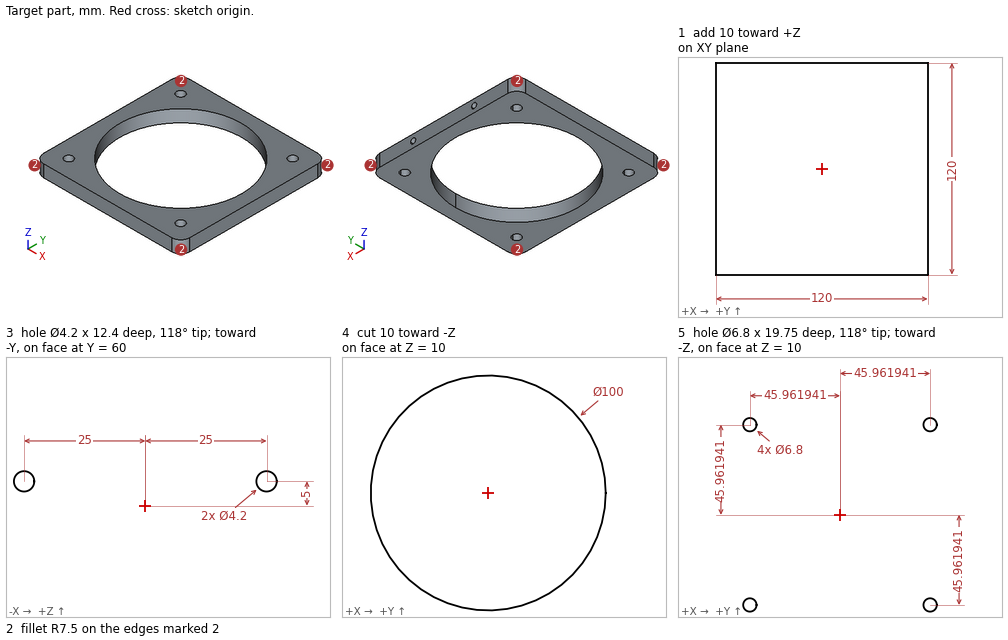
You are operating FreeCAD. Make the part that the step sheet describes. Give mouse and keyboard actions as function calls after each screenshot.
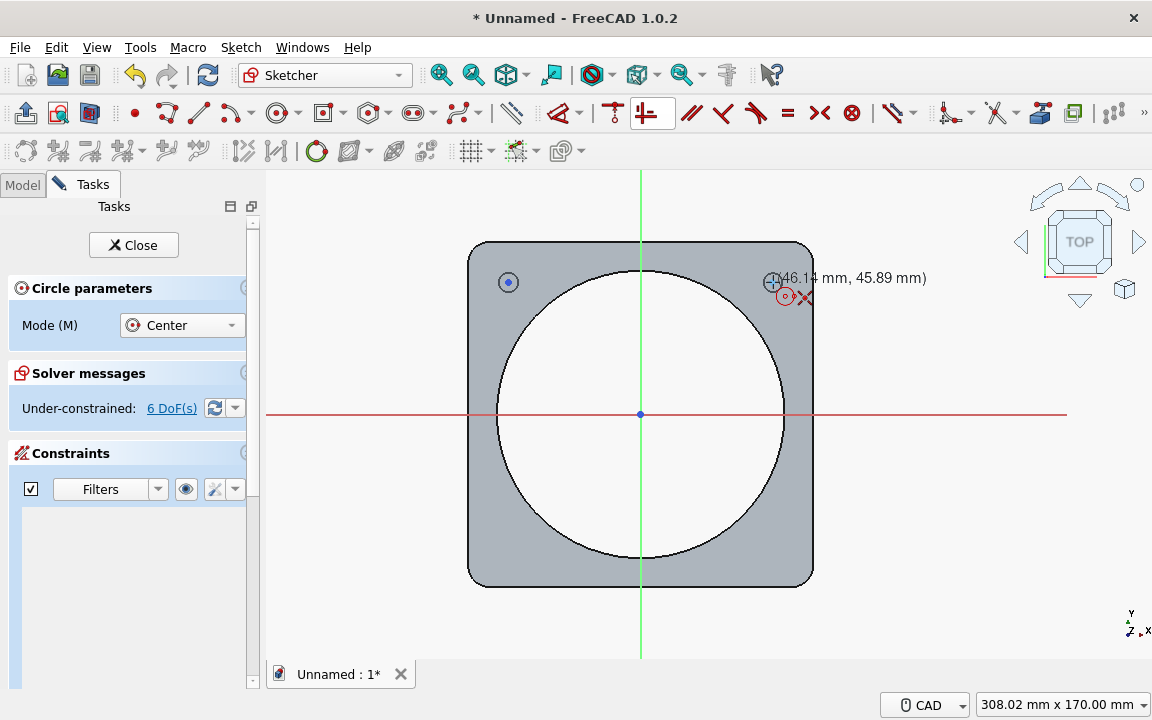
scroll(773, 547, up, 5)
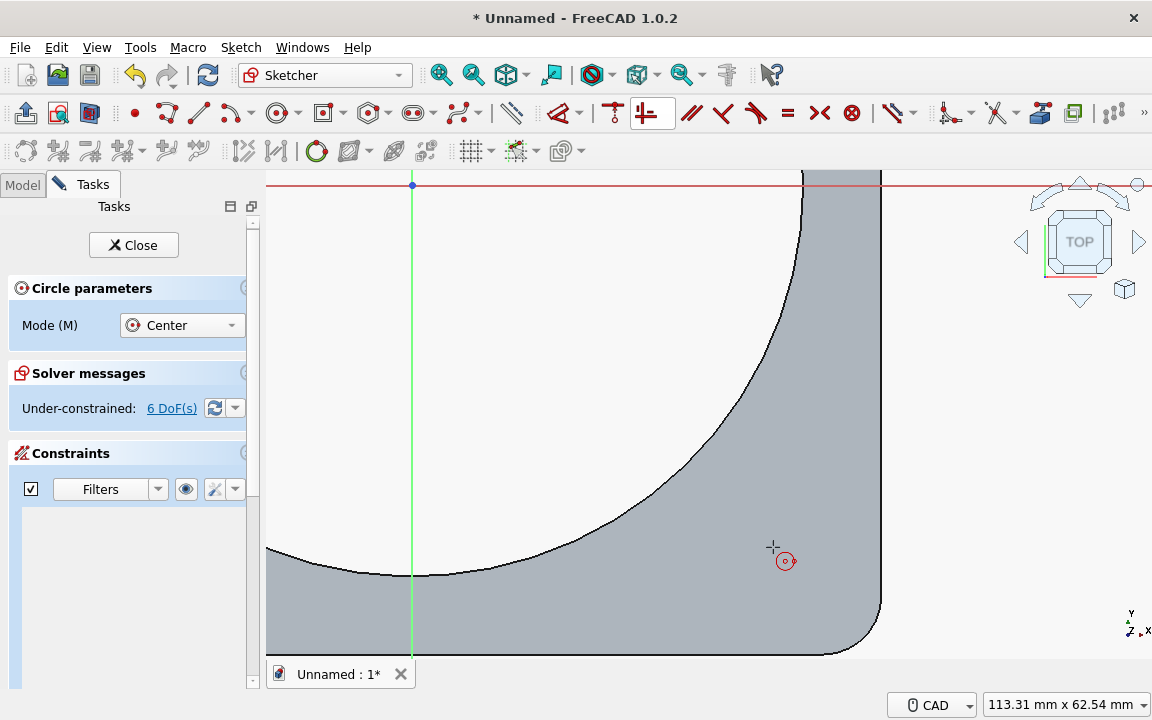
click(772, 545)
click(790, 526)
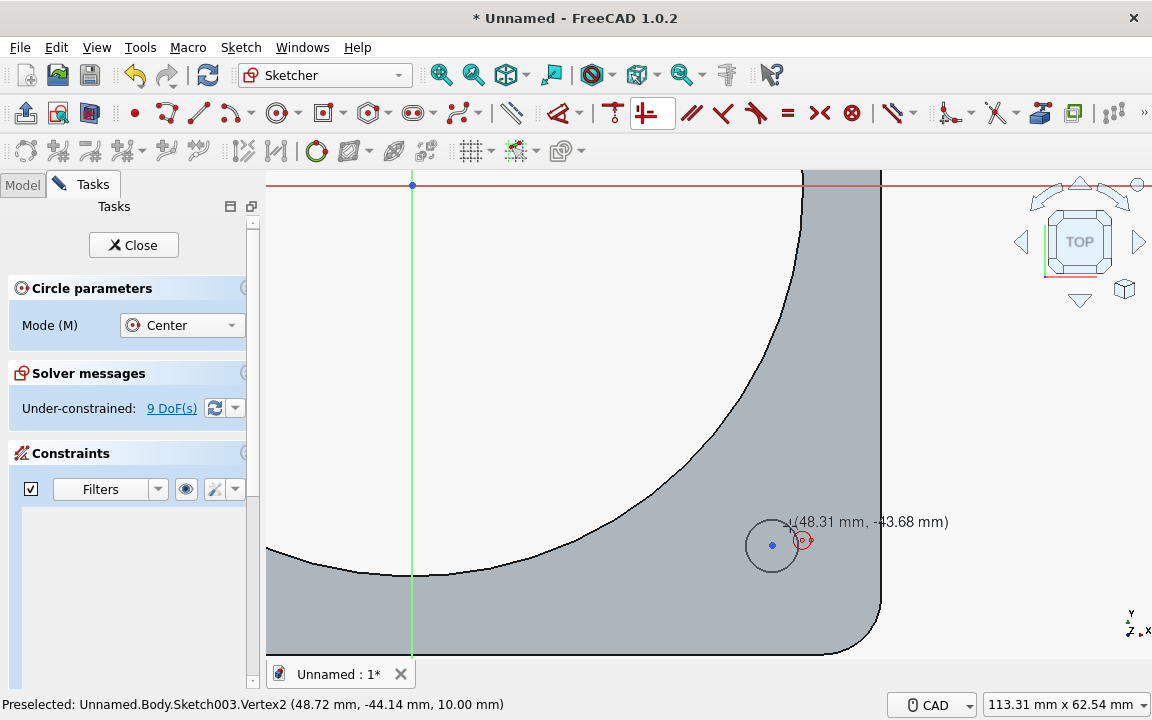
scroll(773, 548, down, 5)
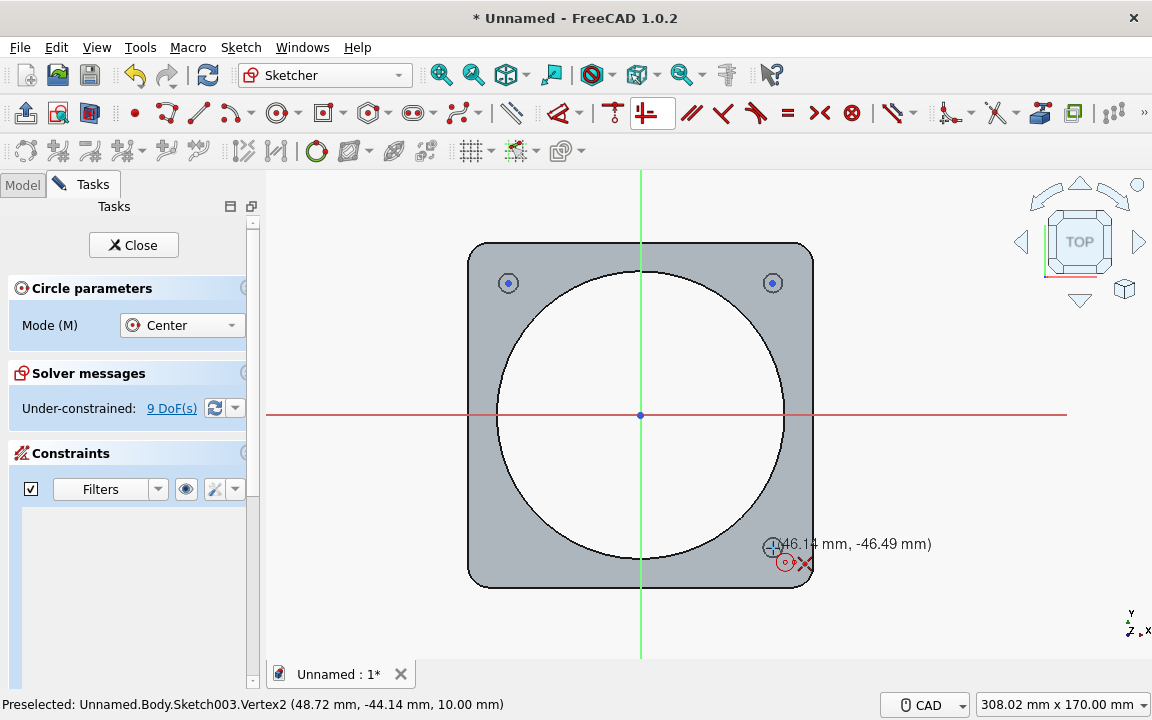
scroll(508, 547, up, 5)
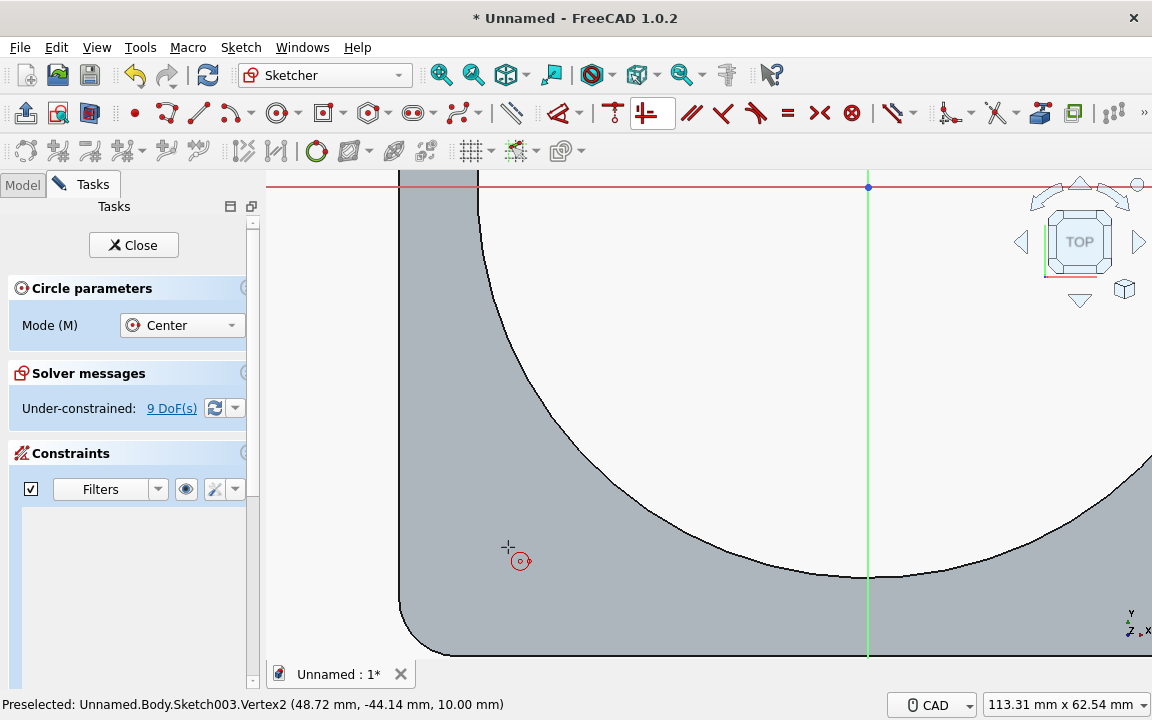
click(509, 547)
click(528, 528)
key(Escape)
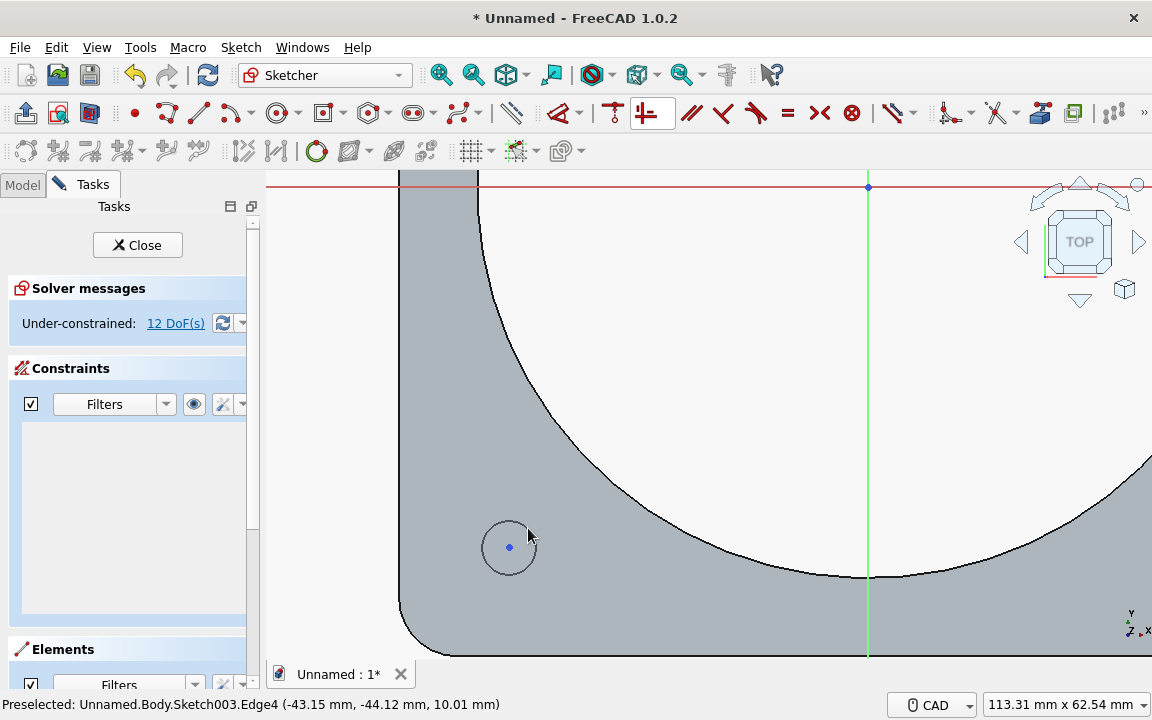
scroll(508, 547, down, 5)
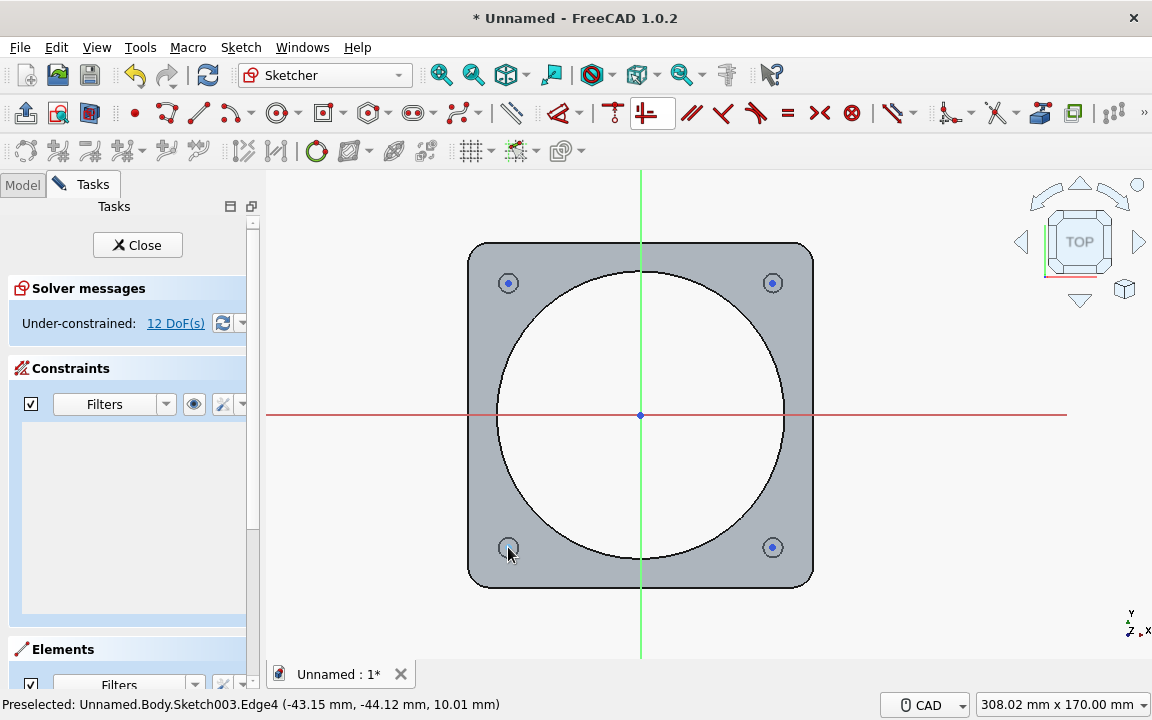
scroll(515, 276, up, 2)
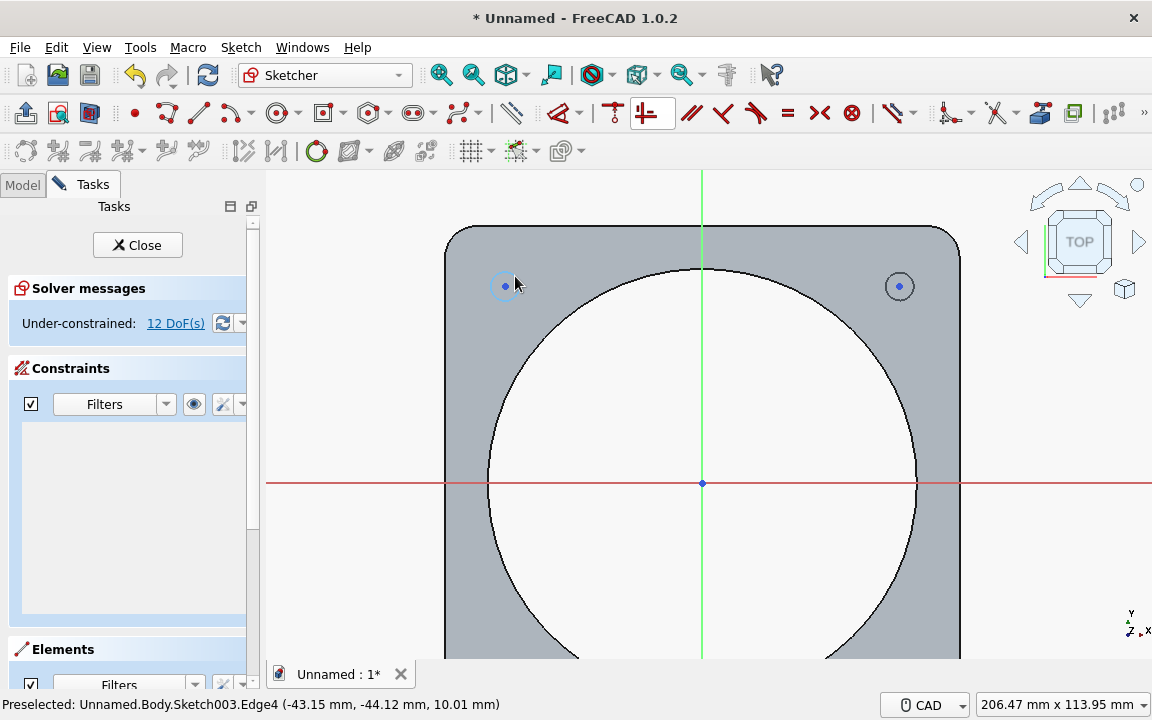
click(515, 276)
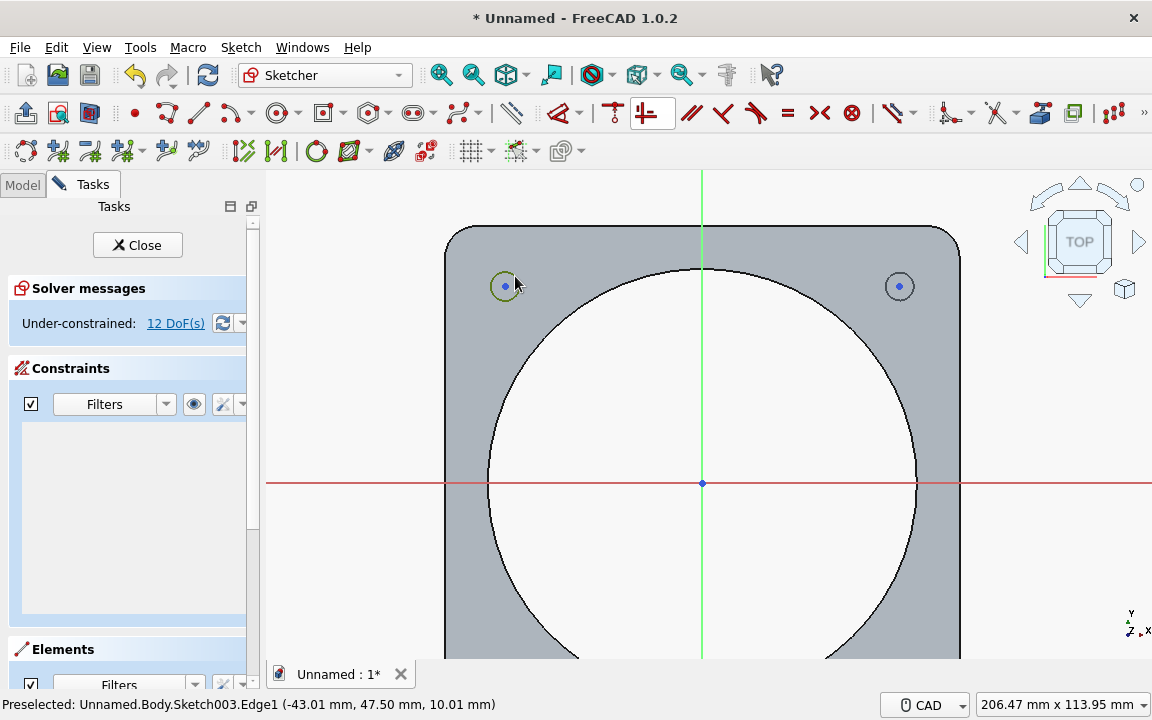
click(910, 277)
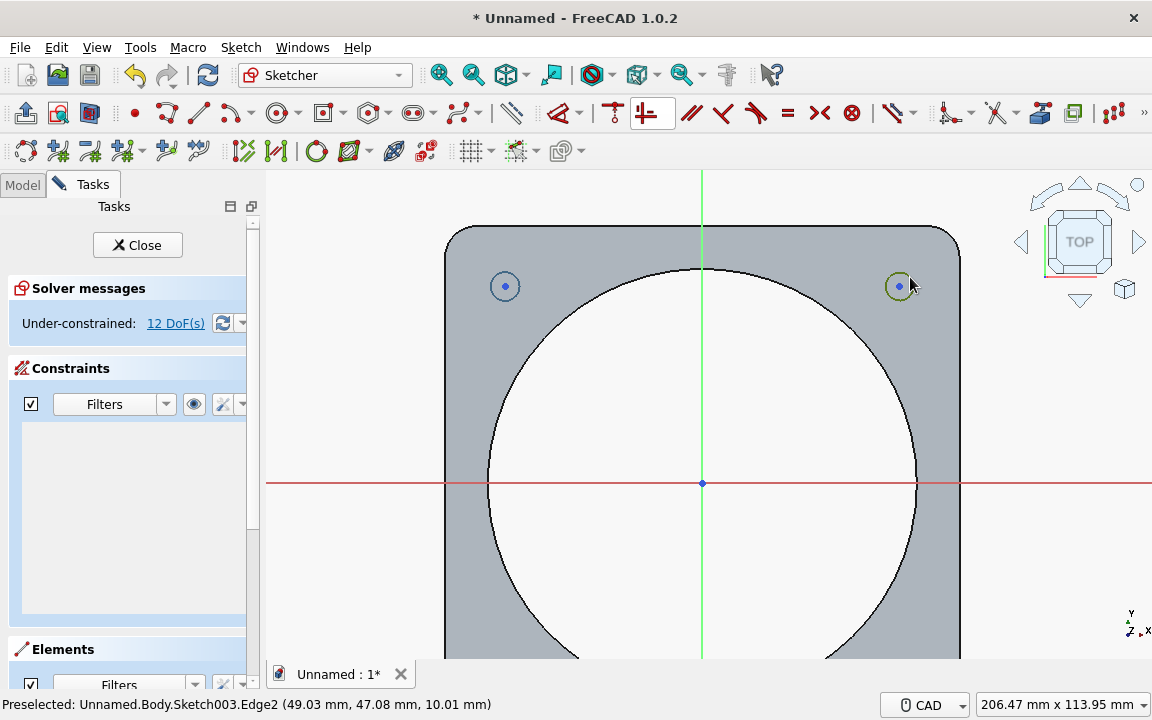
scroll(515, 274, down, 2)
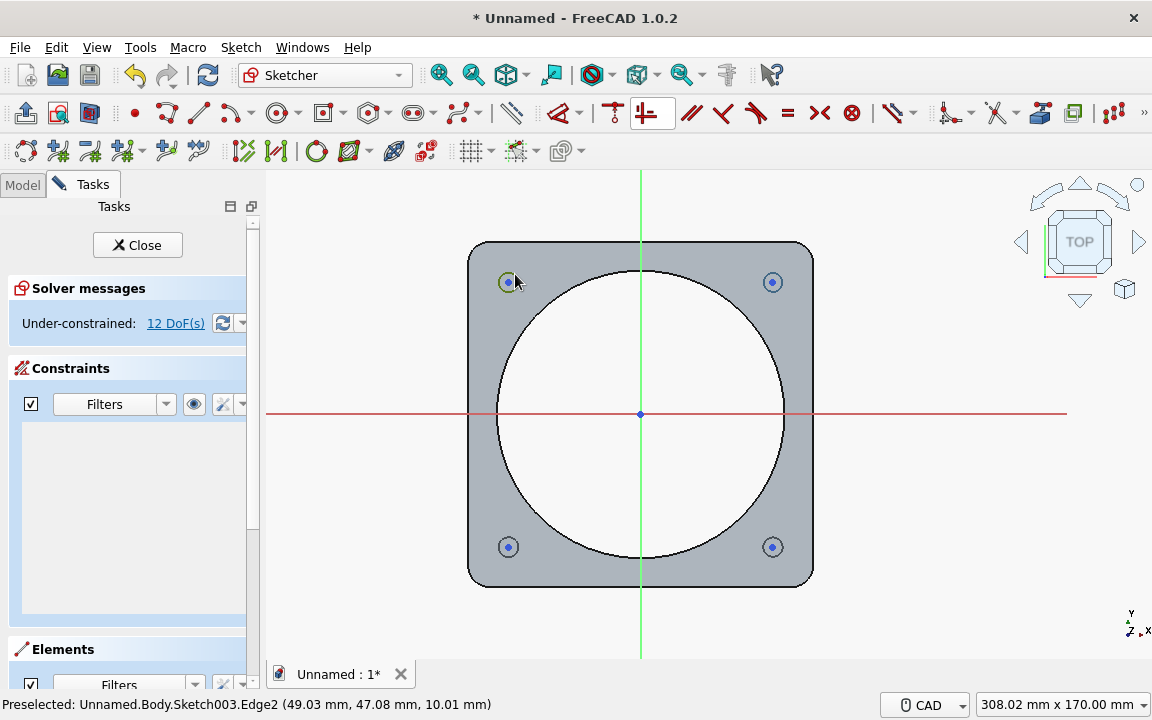
scroll(780, 540, up, 2)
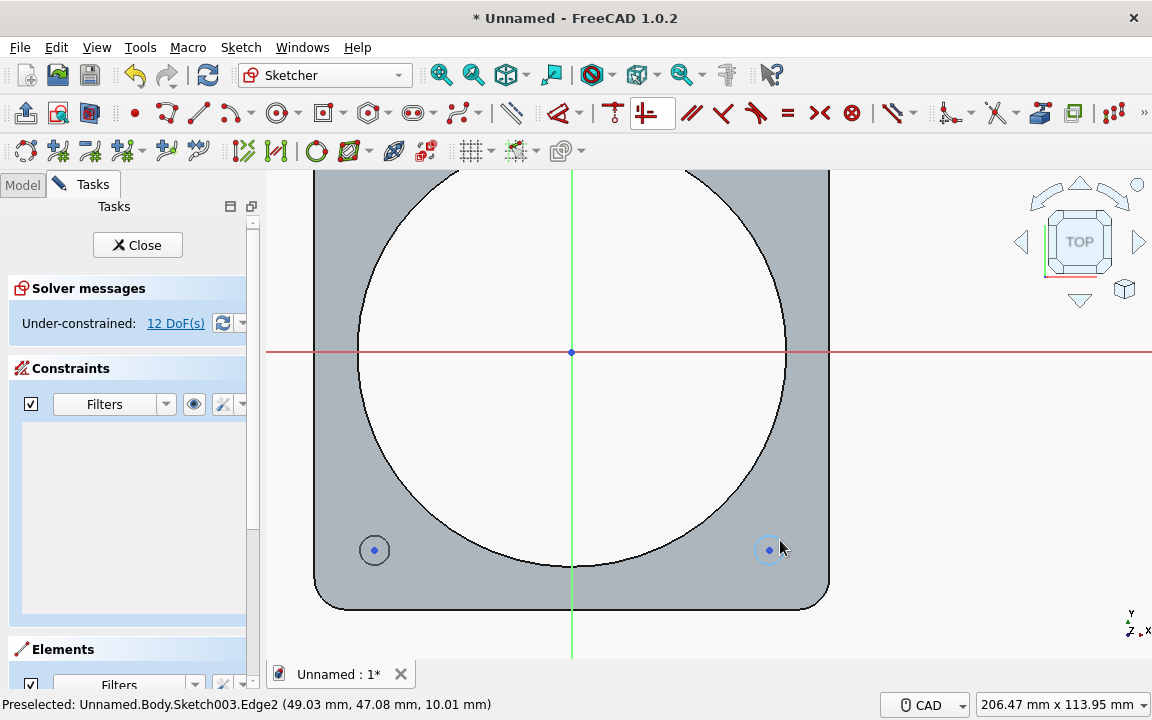
click(779, 540)